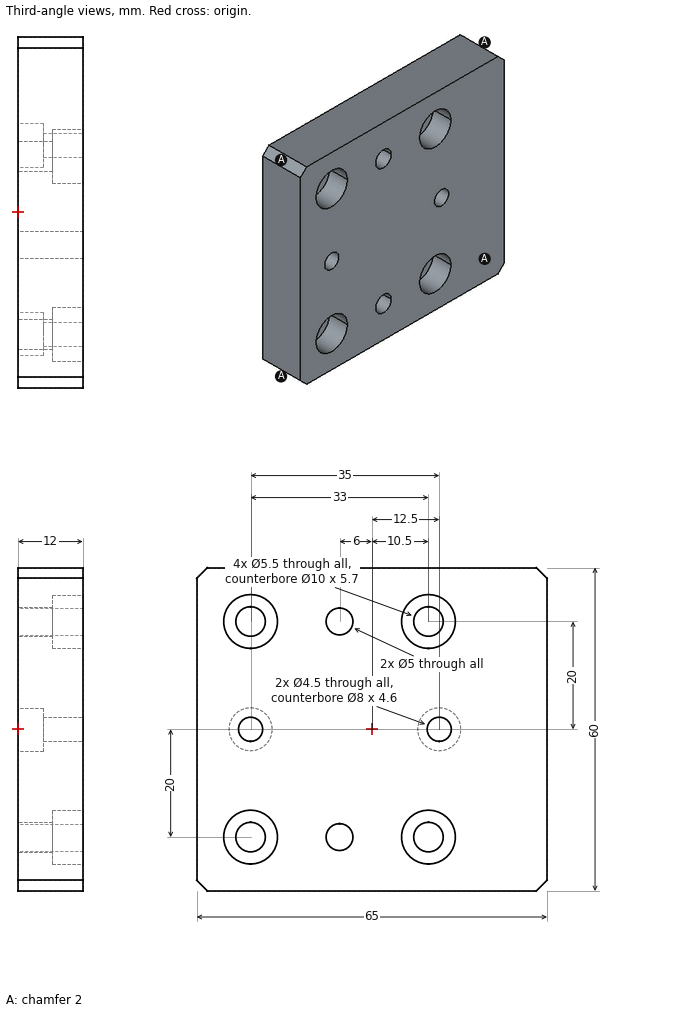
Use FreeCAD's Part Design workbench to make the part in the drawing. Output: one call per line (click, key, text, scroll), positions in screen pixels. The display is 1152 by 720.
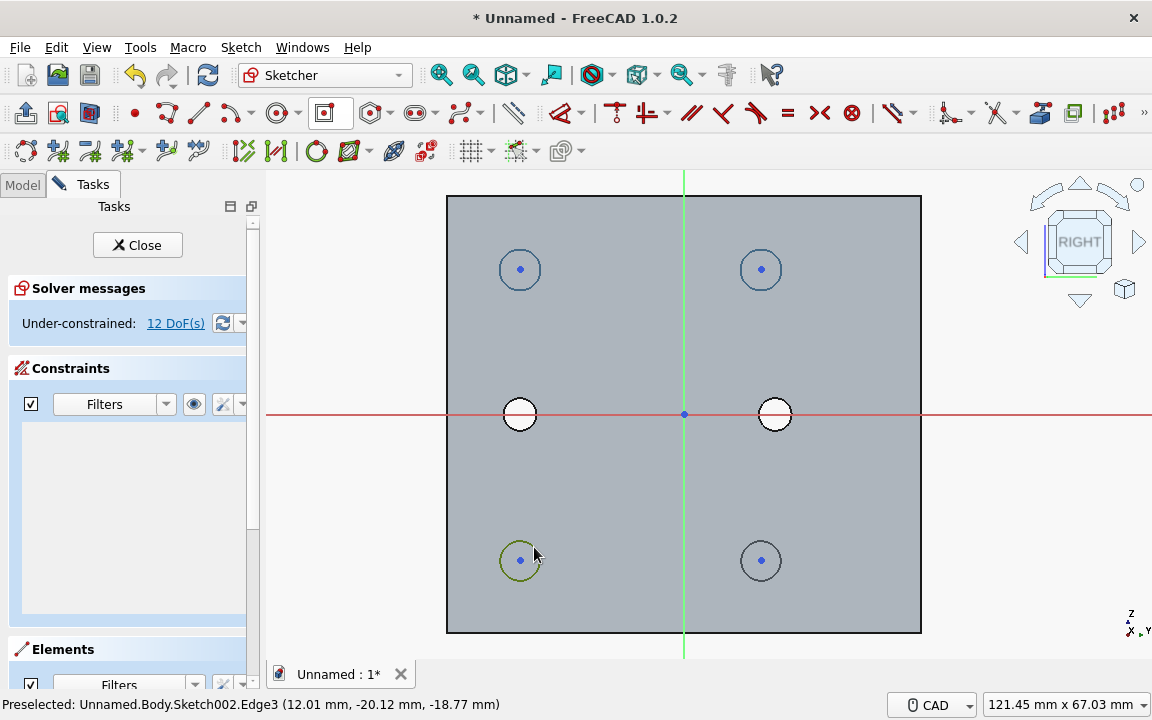
click(775, 547)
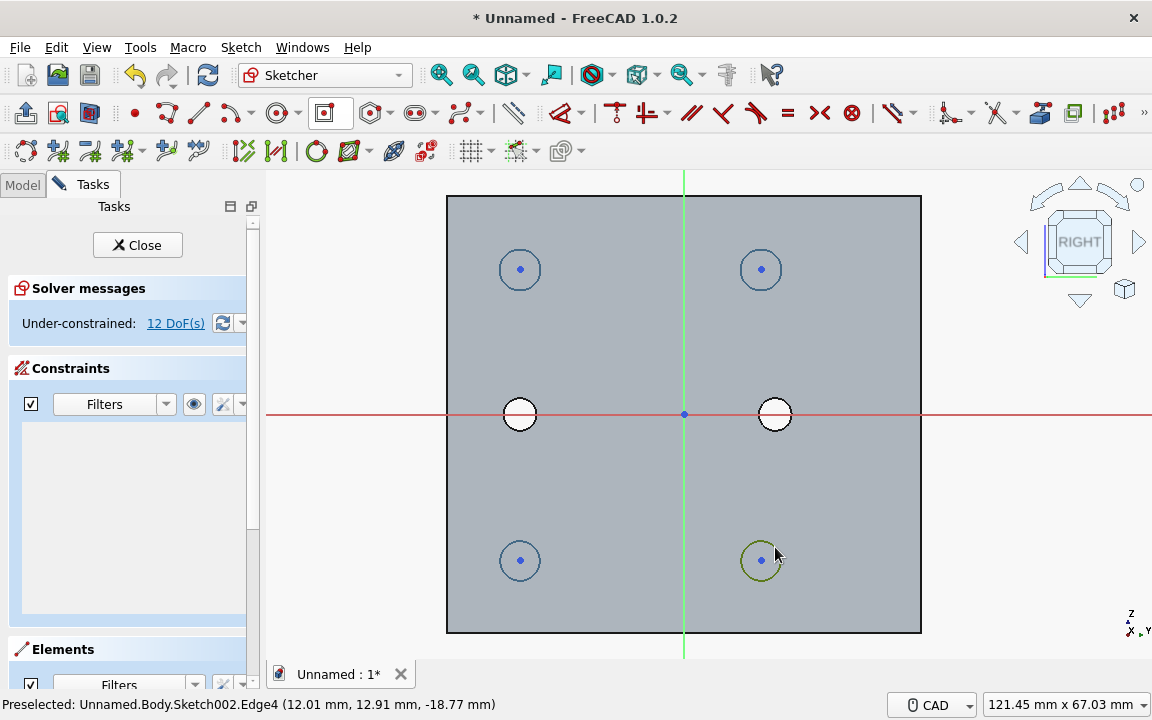
click(788, 114)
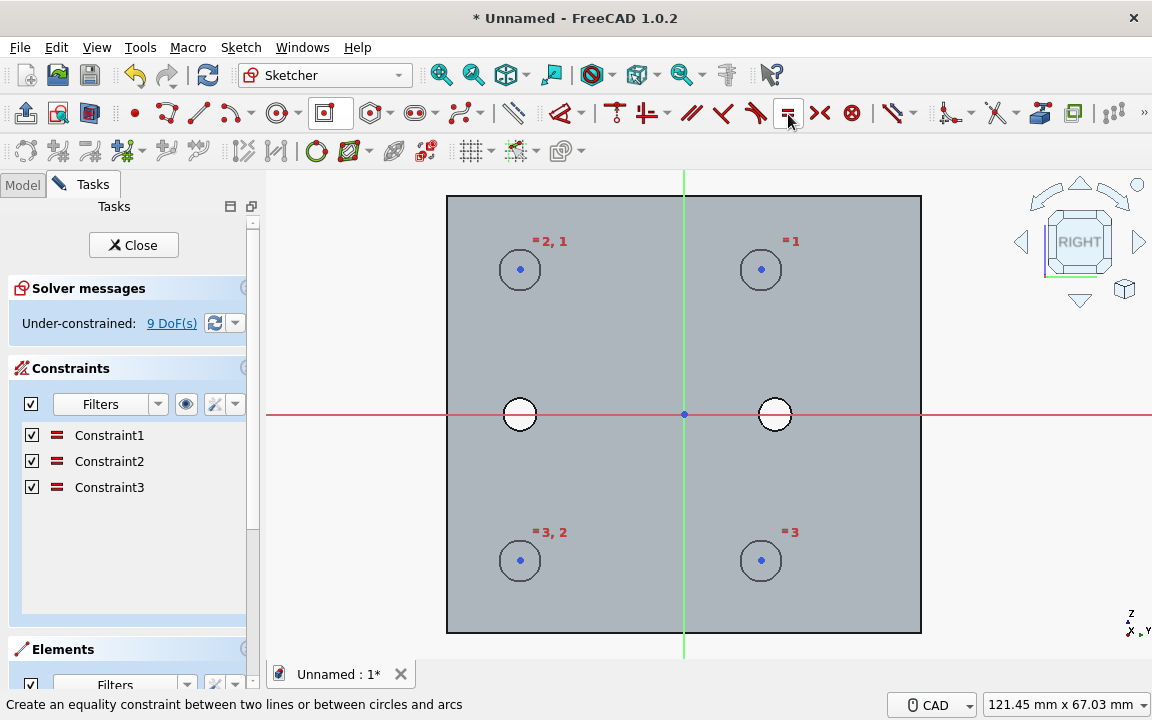
click(761, 270)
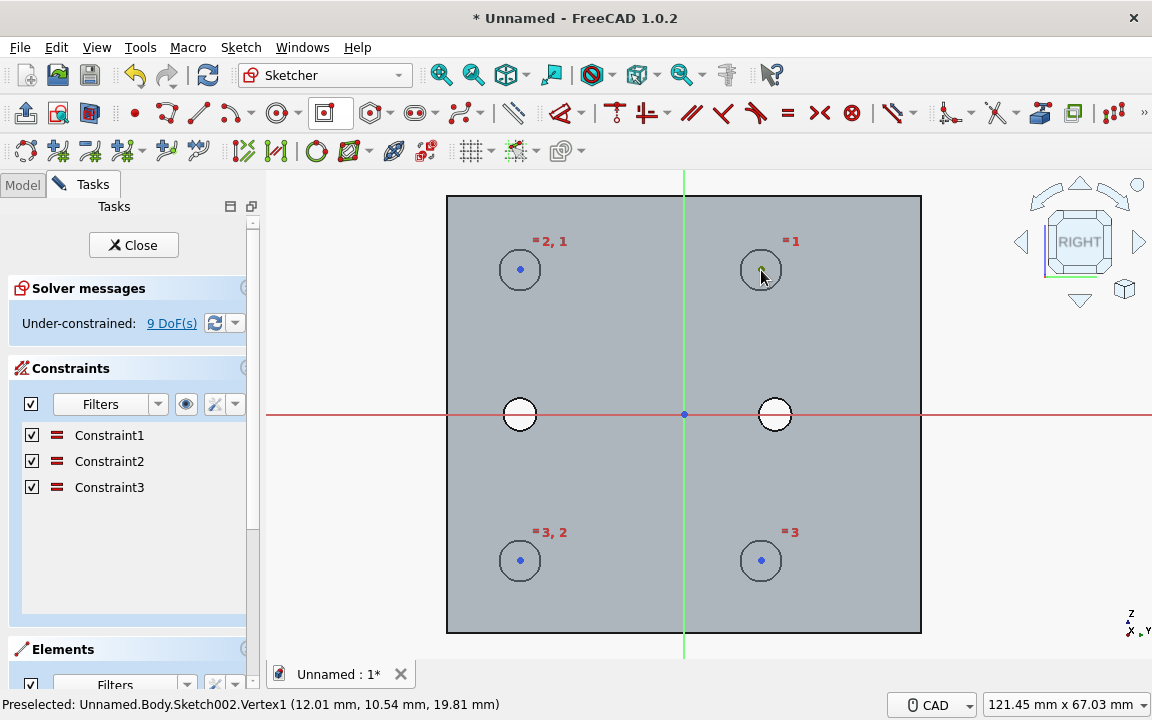
click(520, 270)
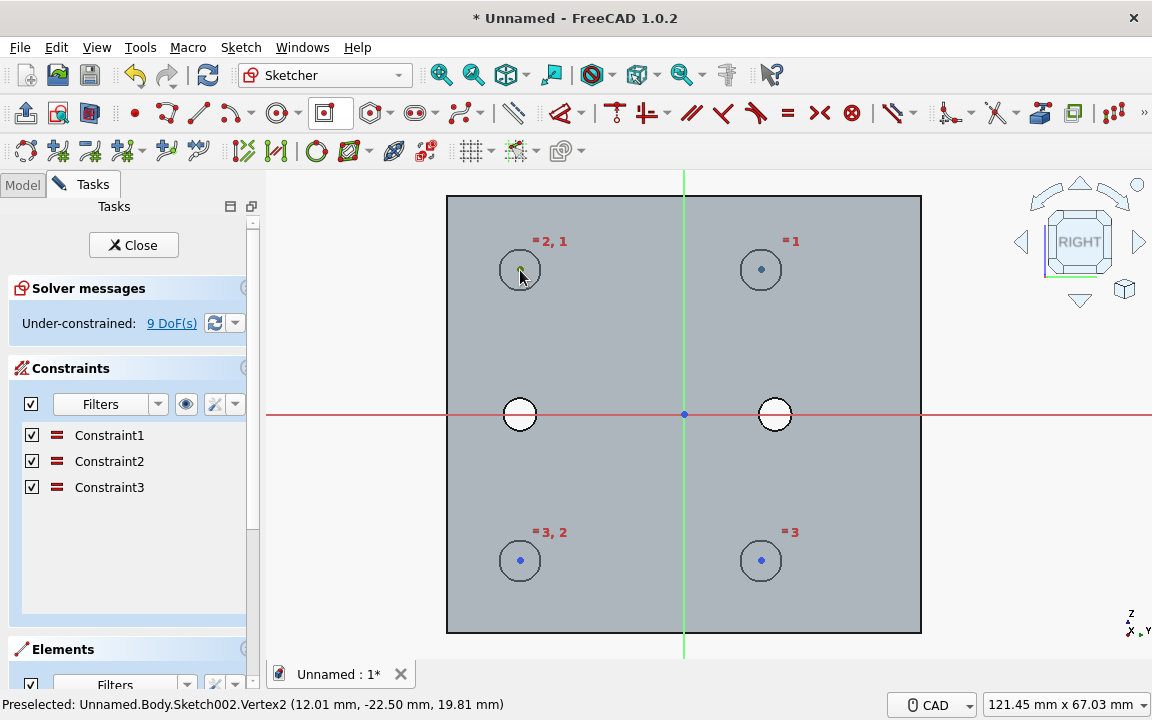
click(670, 114)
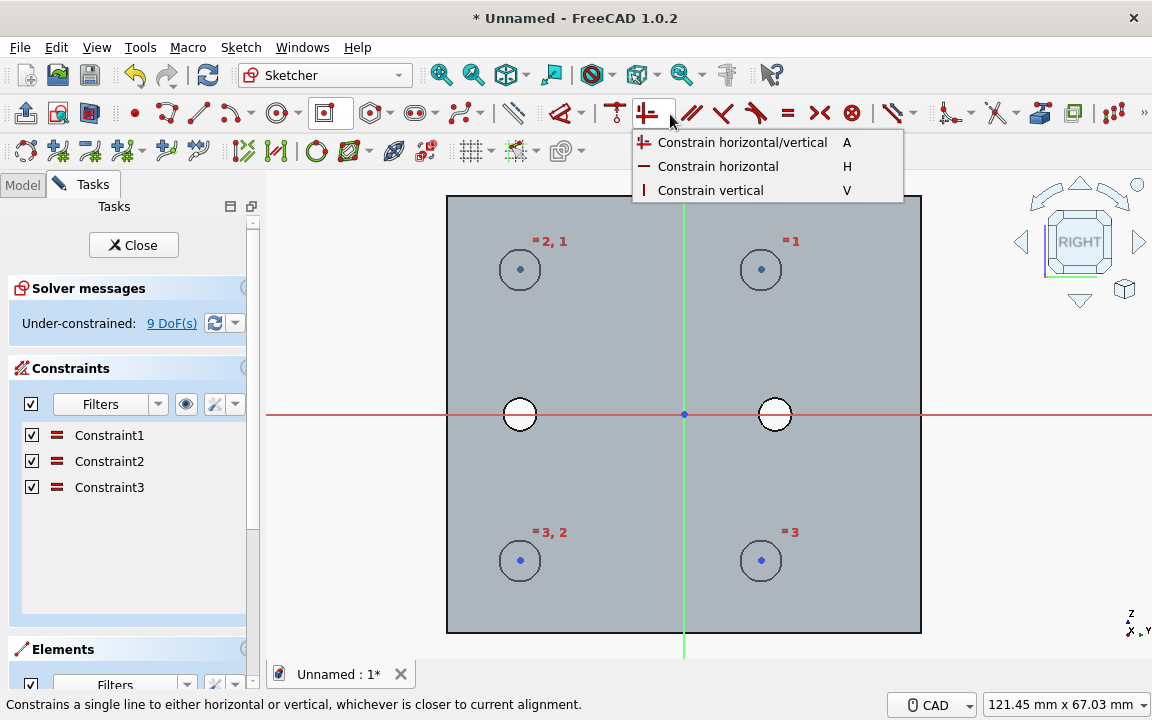
click(768, 166)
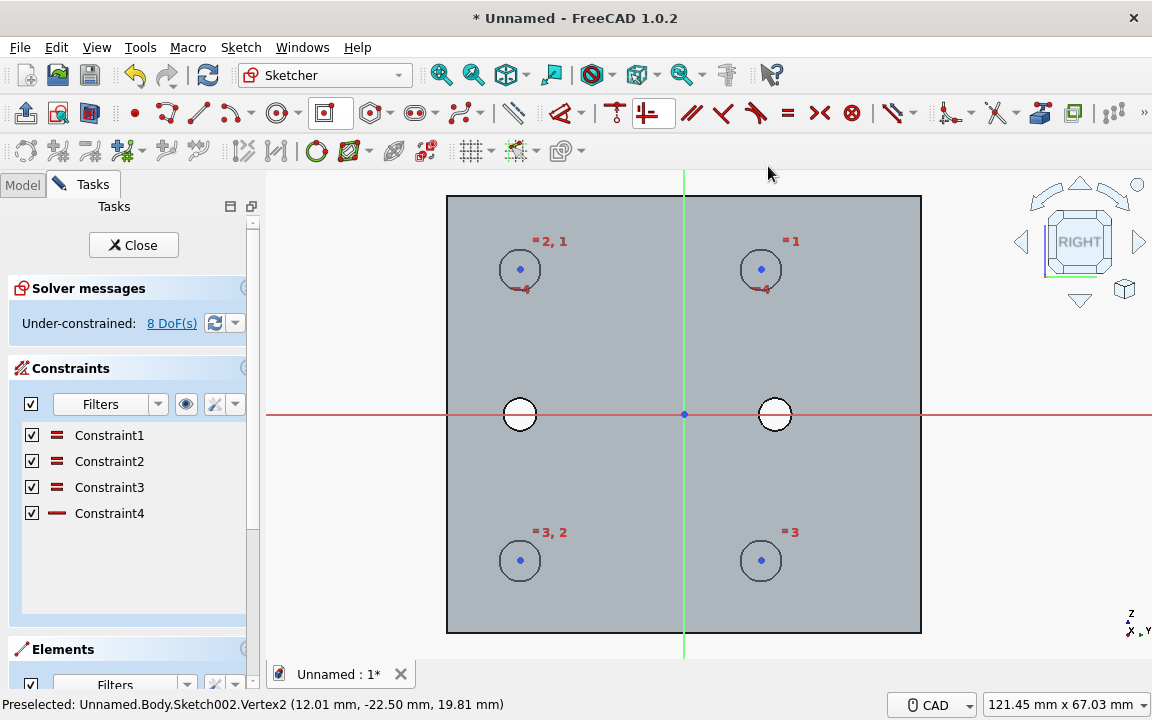
click(520, 270)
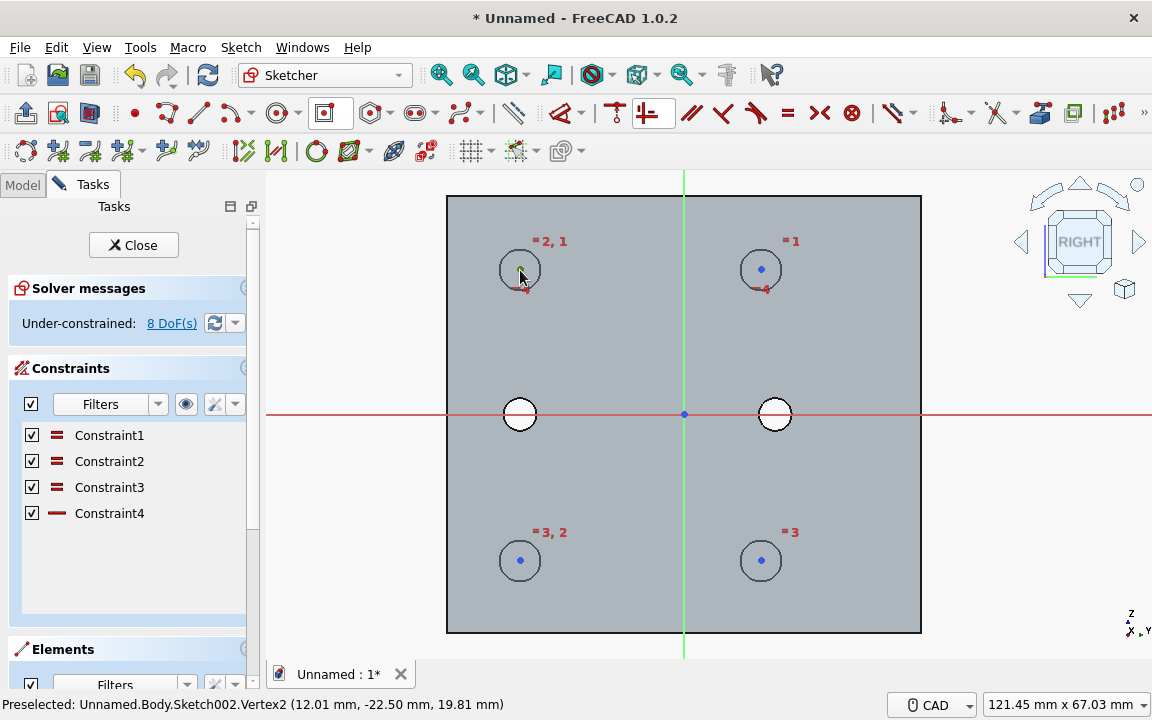
click(520, 561)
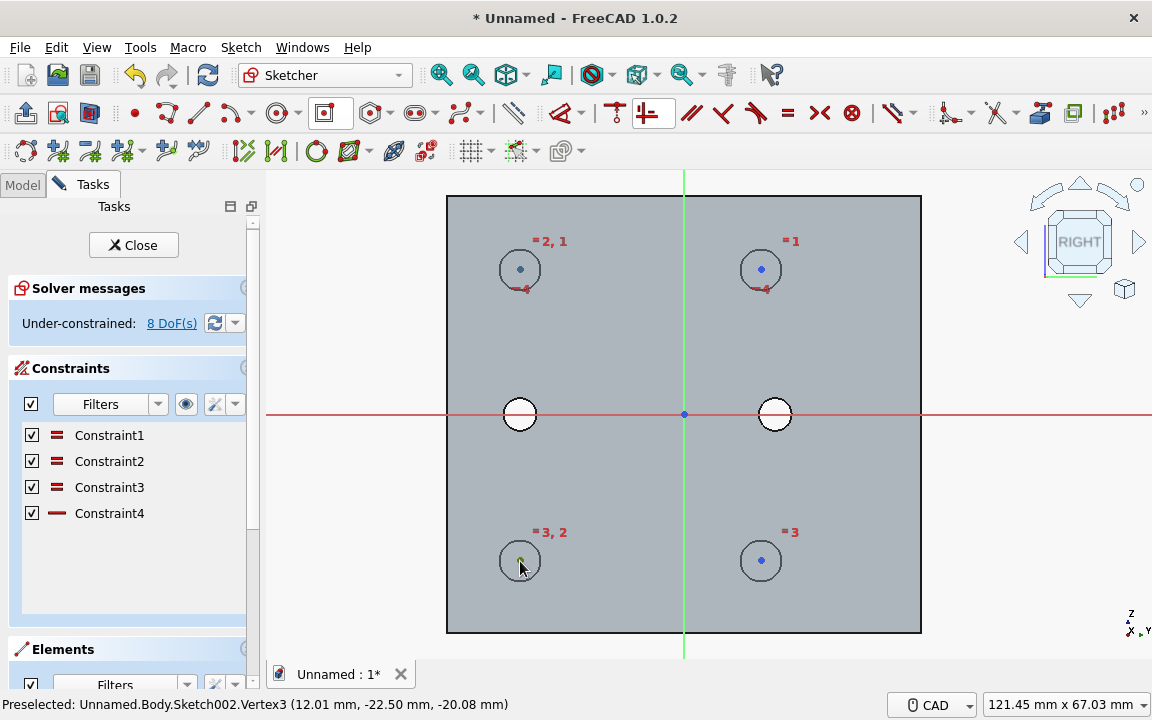
click(670, 114)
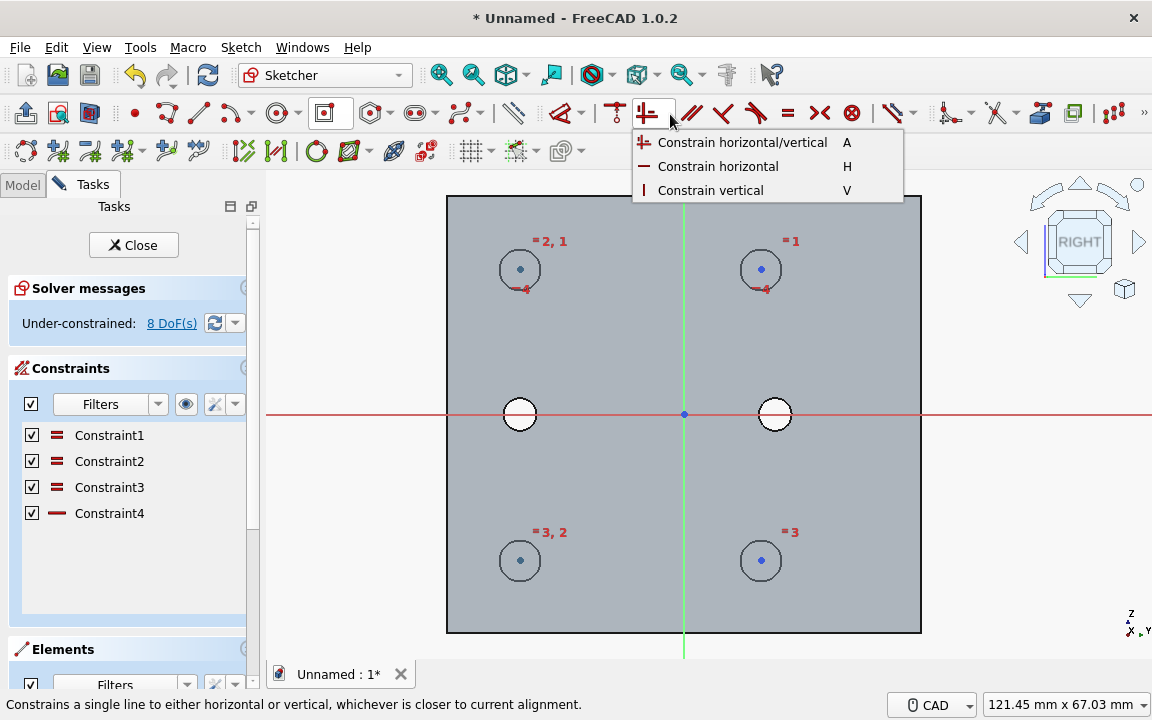
click(768, 190)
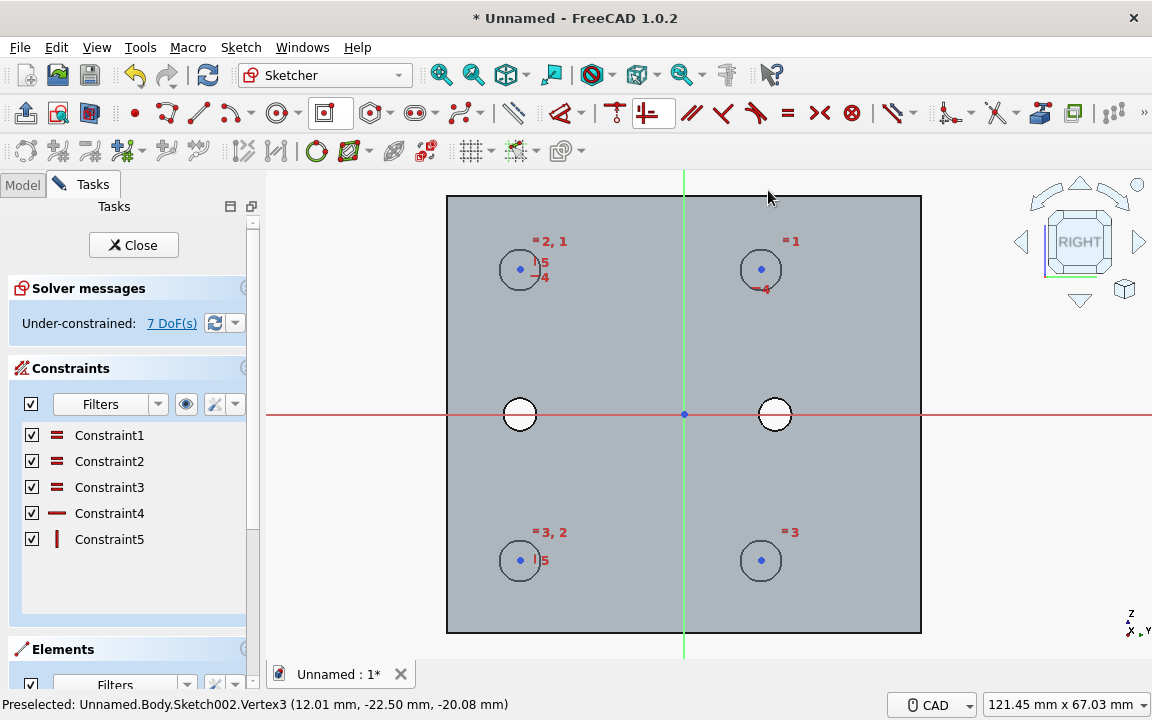
click(761, 270)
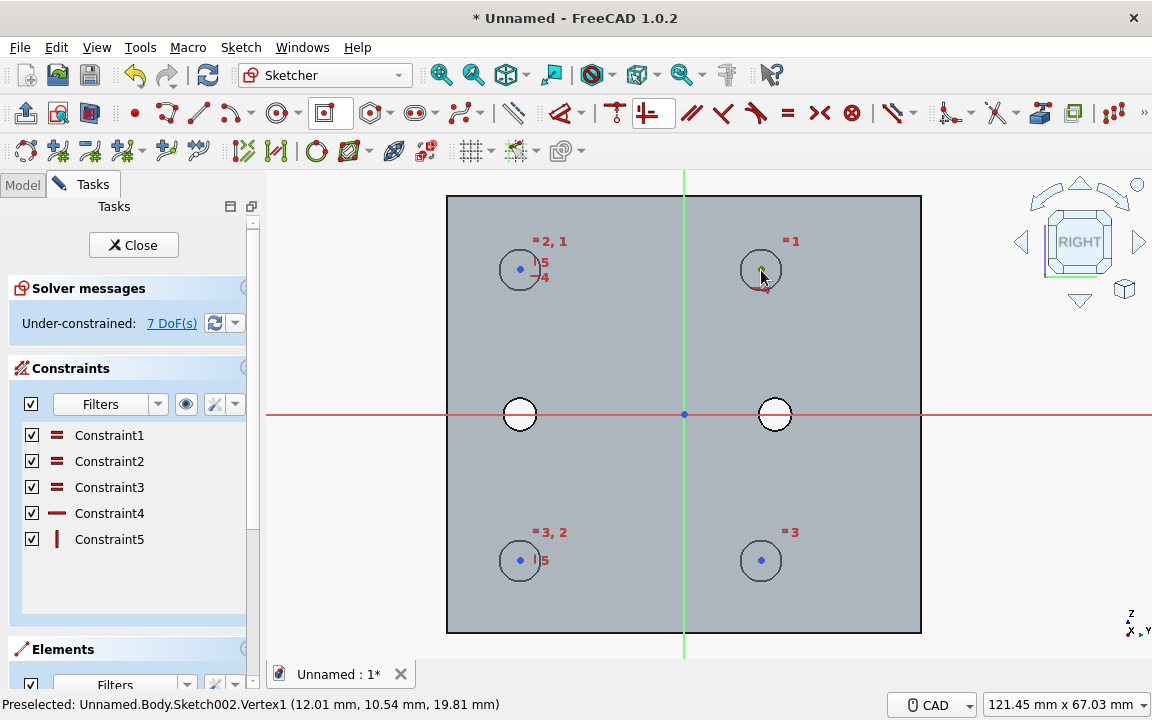
click(761, 561)